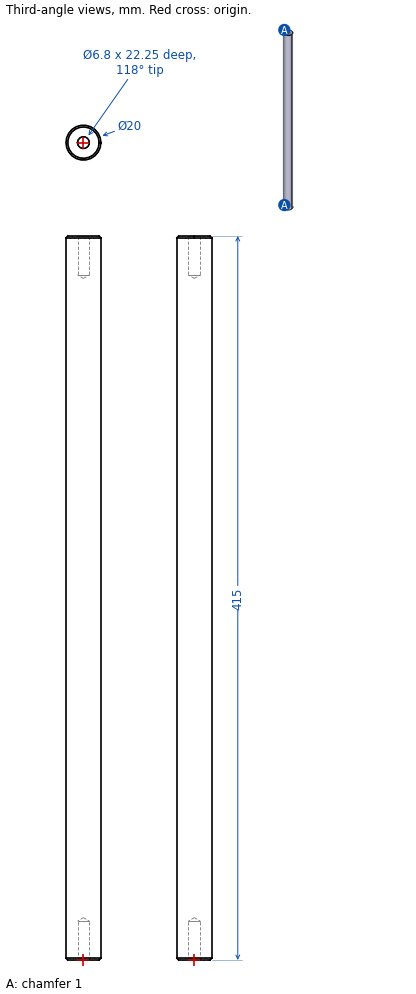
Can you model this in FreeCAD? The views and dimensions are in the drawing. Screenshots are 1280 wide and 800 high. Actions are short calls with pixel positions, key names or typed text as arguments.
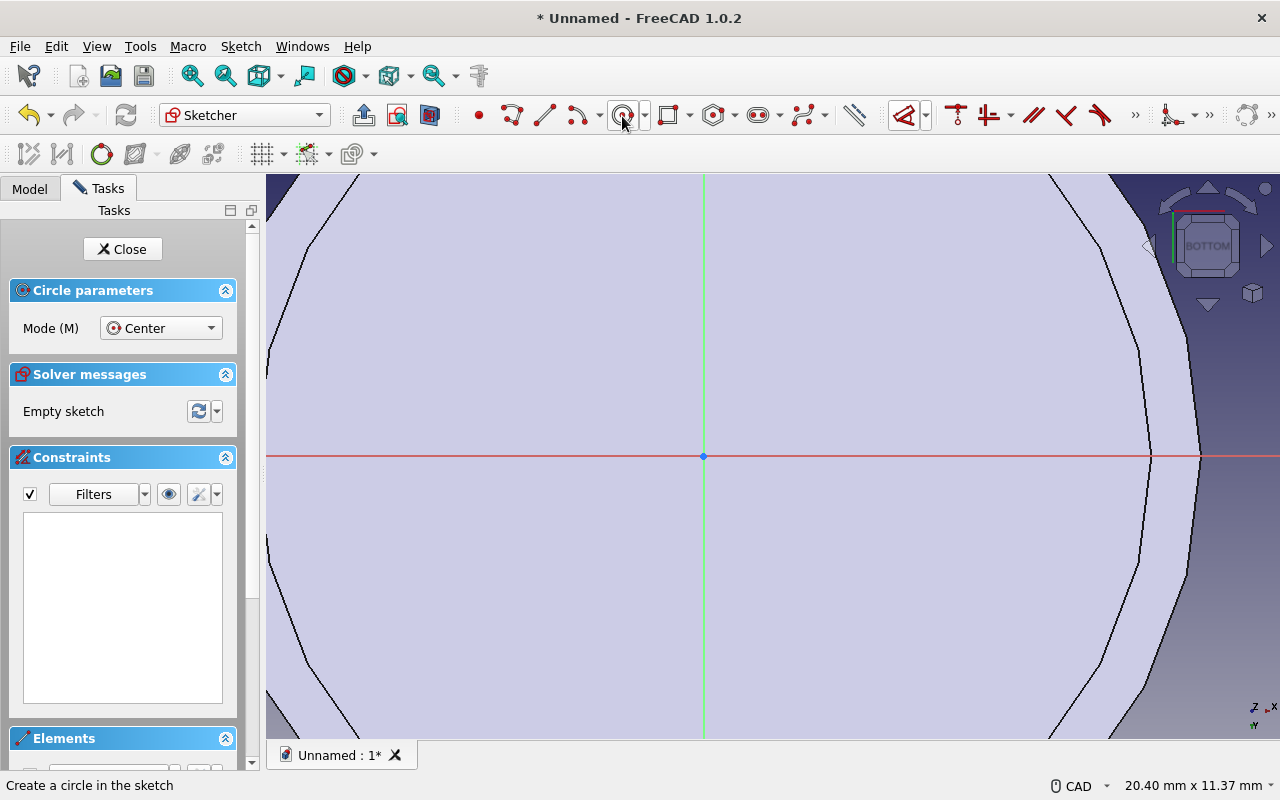
click(704, 456)
click(824, 337)
key(Escape)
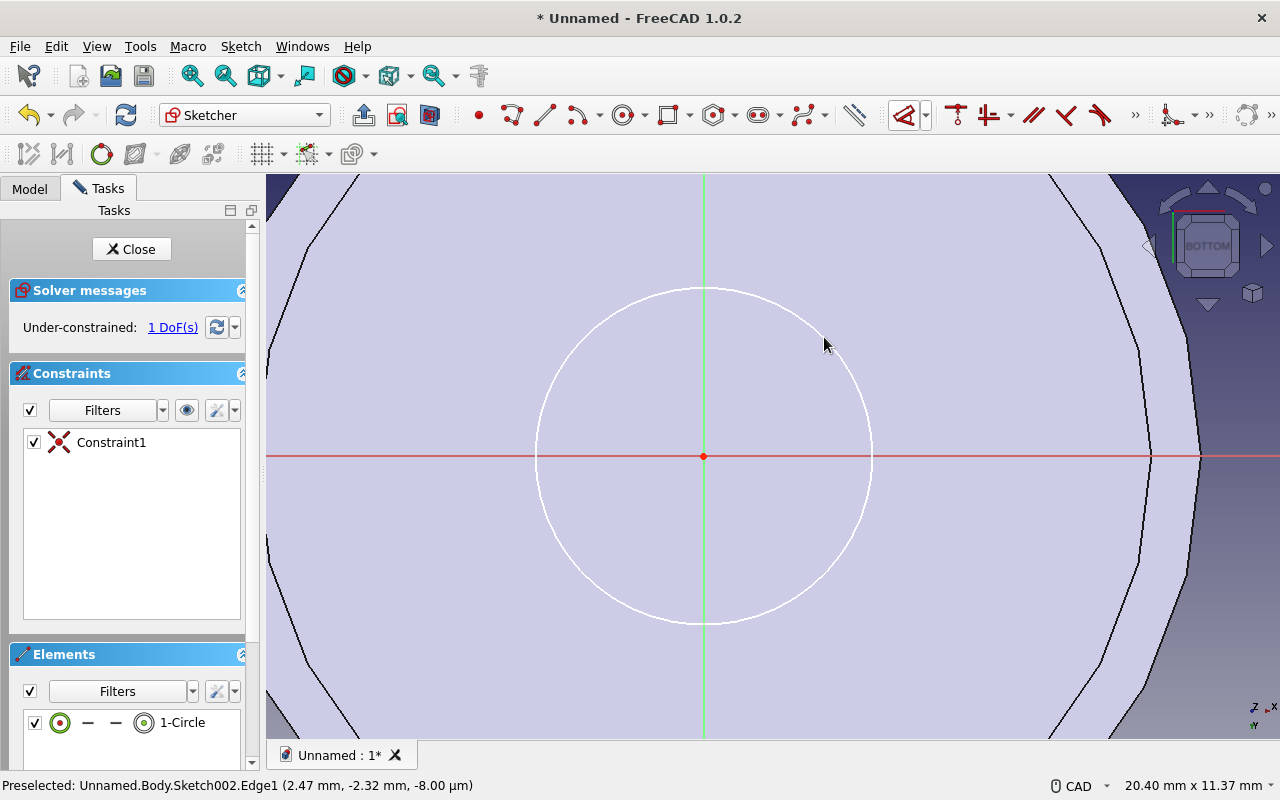
click(823, 337)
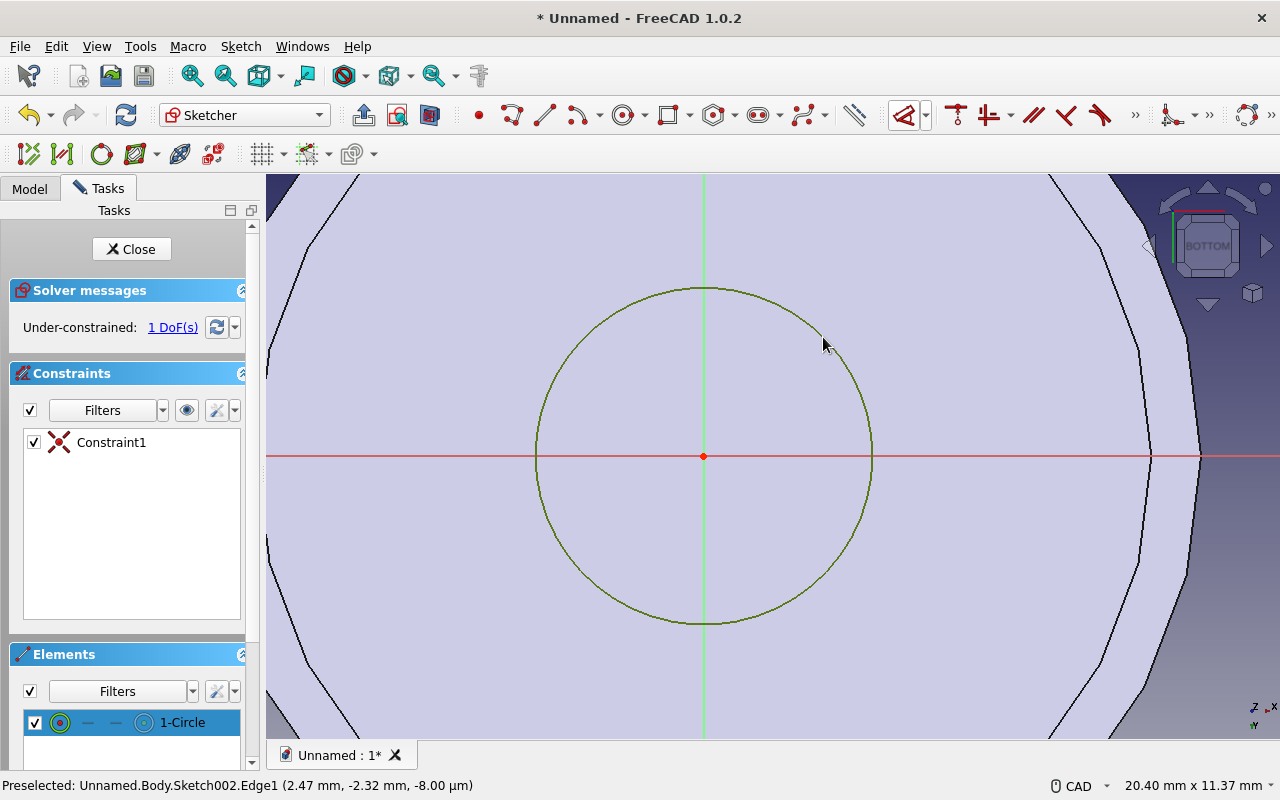
click(926, 116)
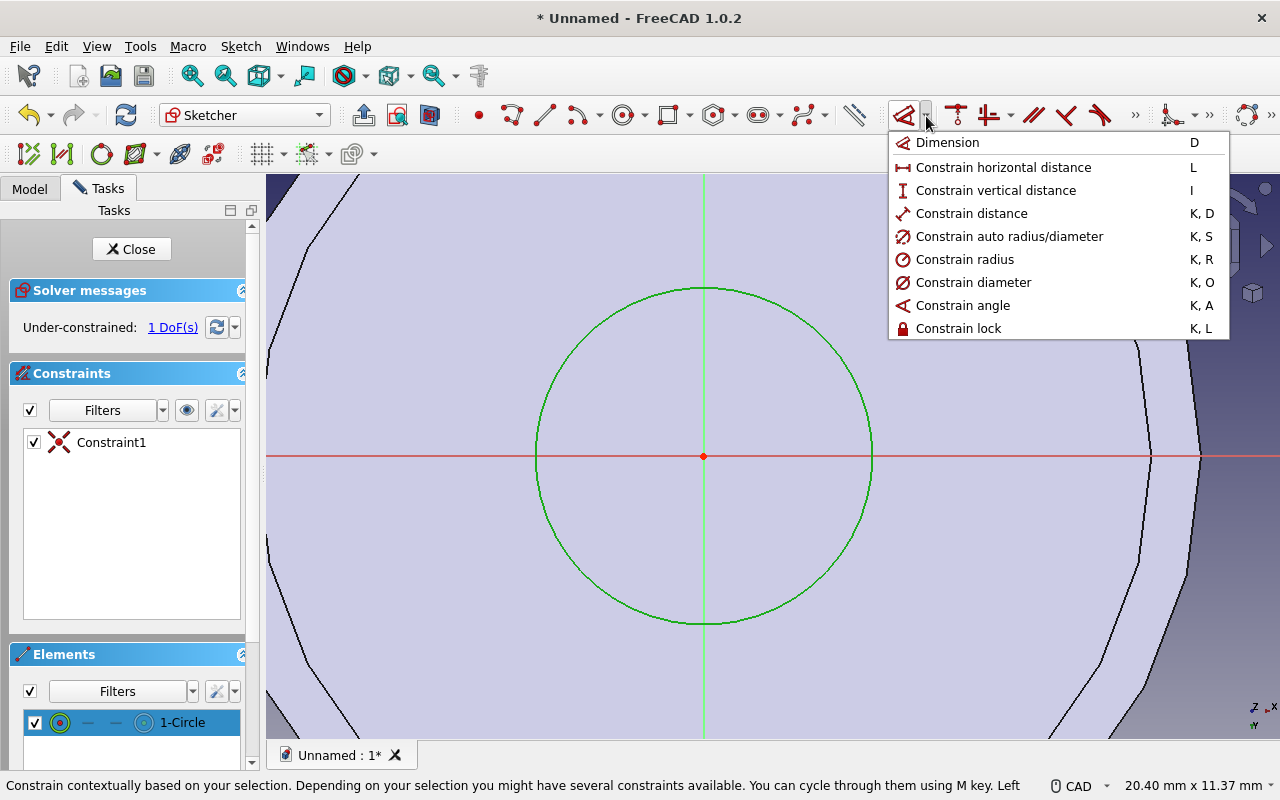
click(1059, 282)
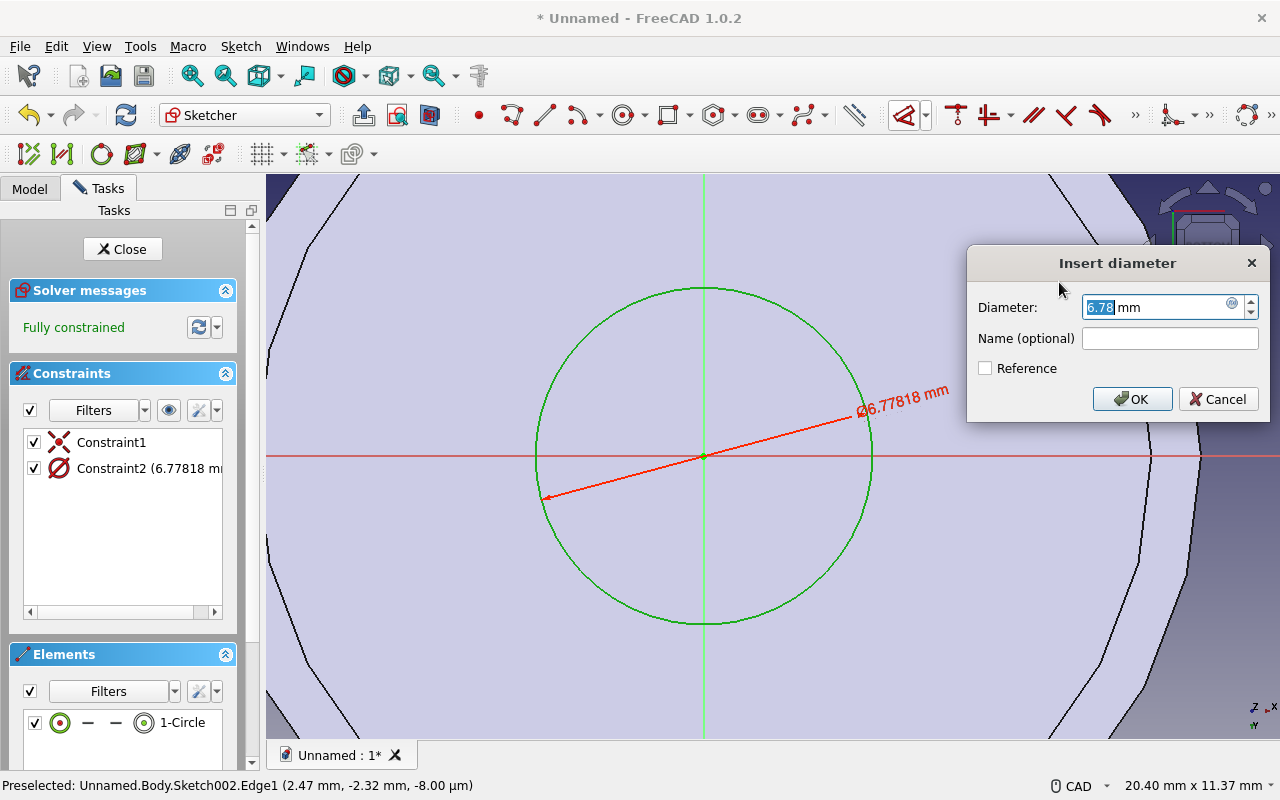
text(6.8)
key(Return)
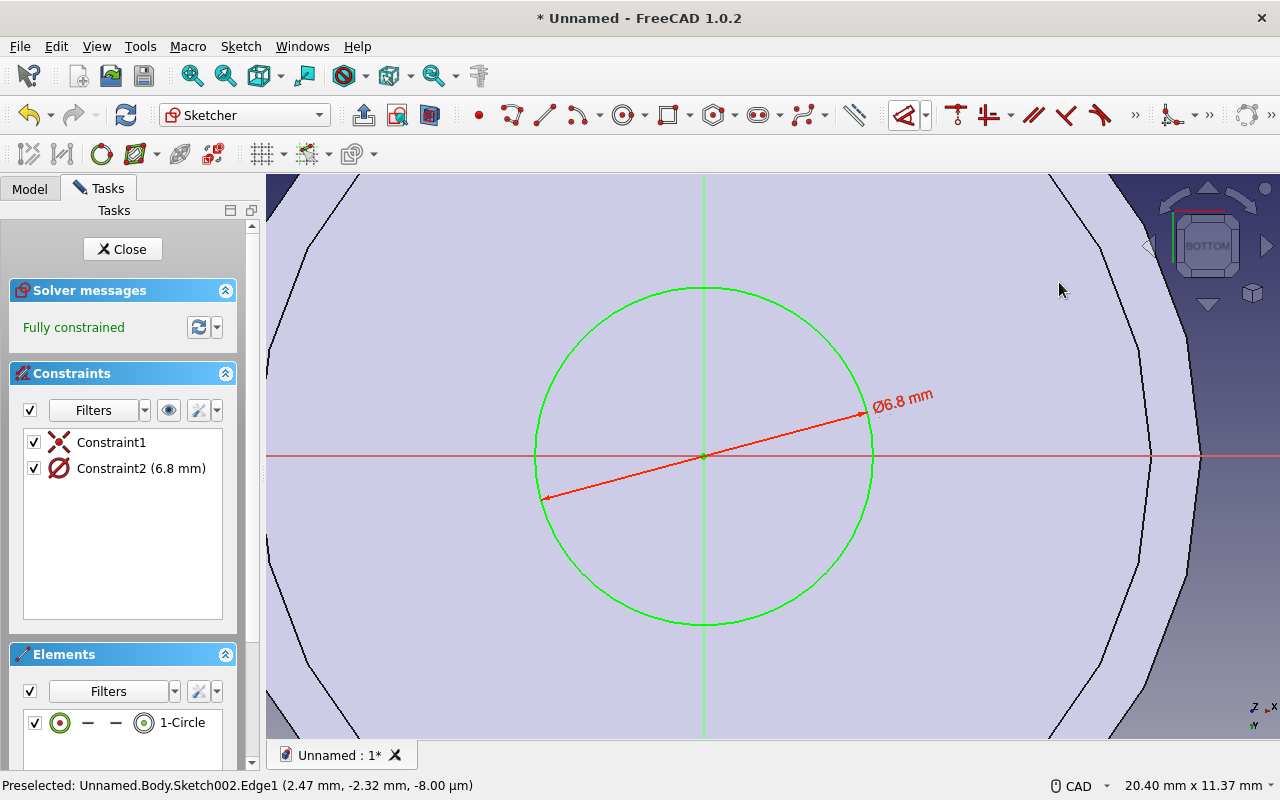
click(123, 249)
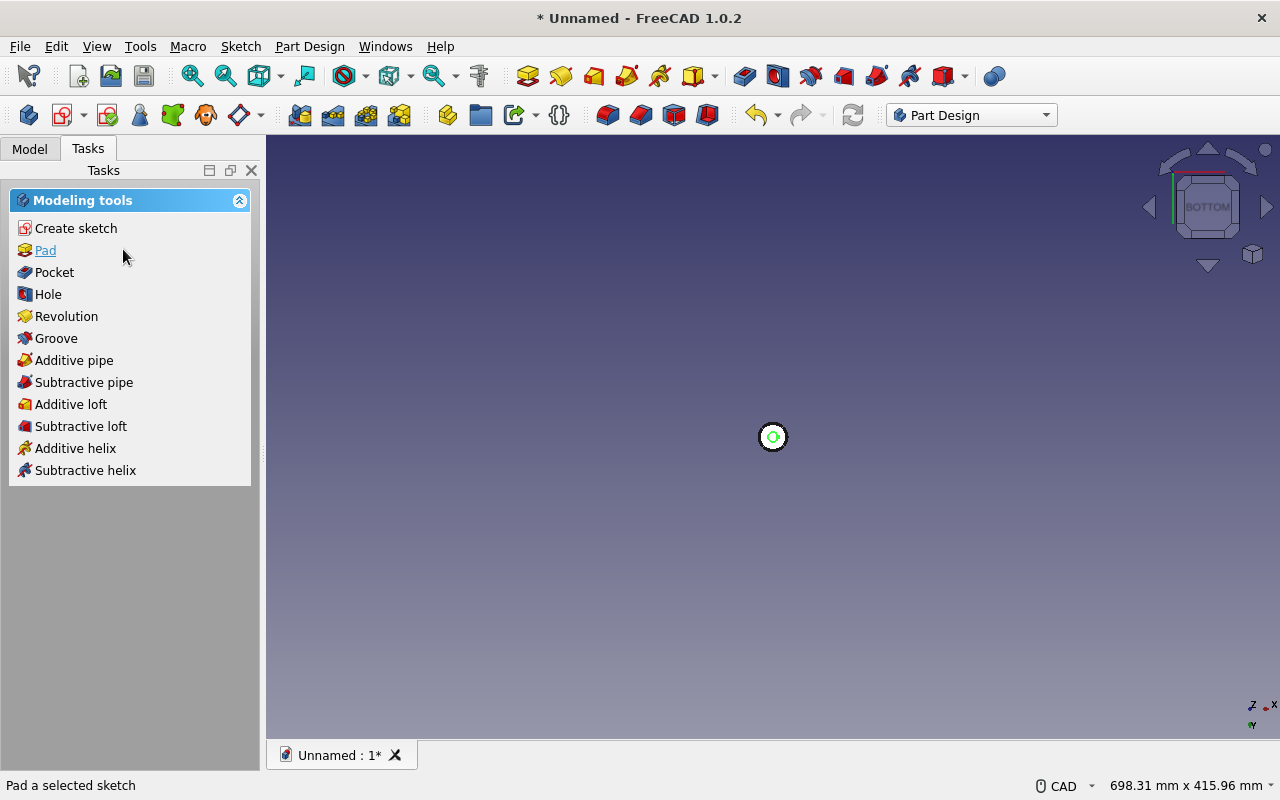
click(778, 76)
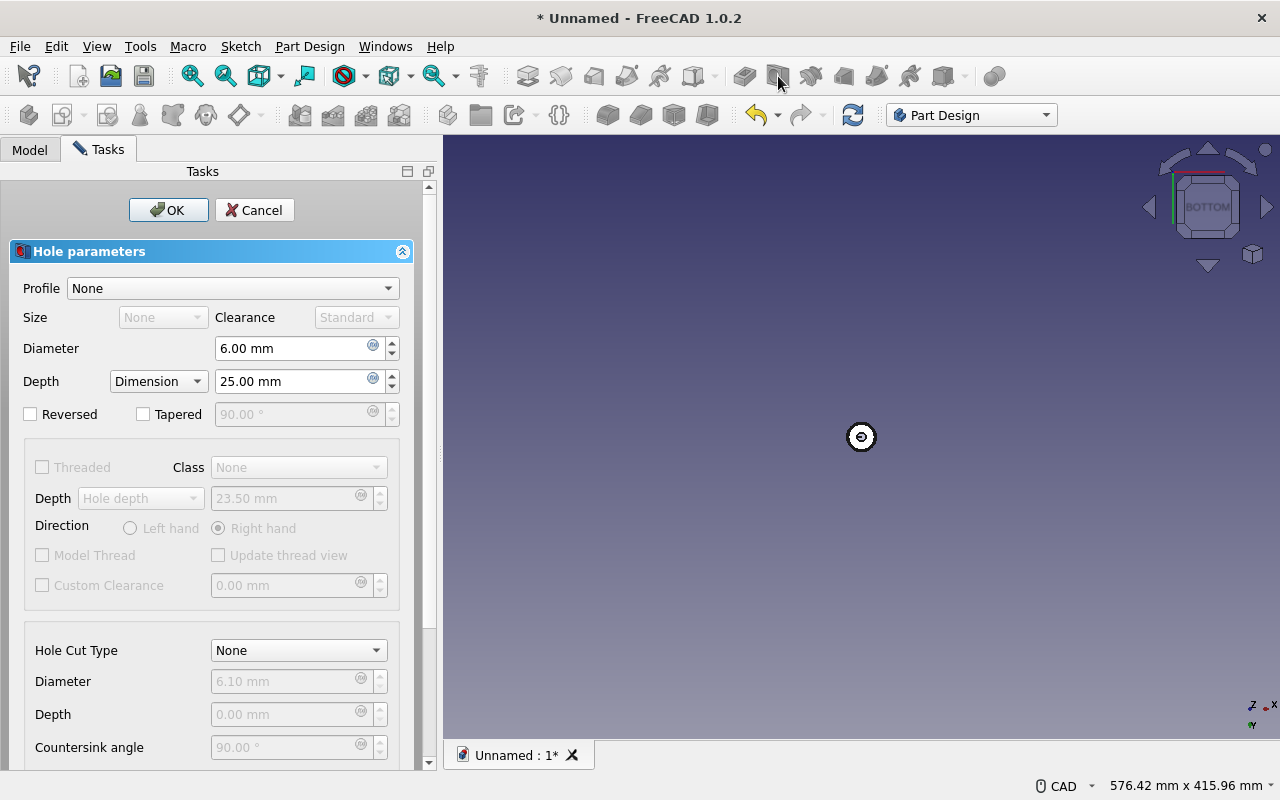
triple_click(300, 348)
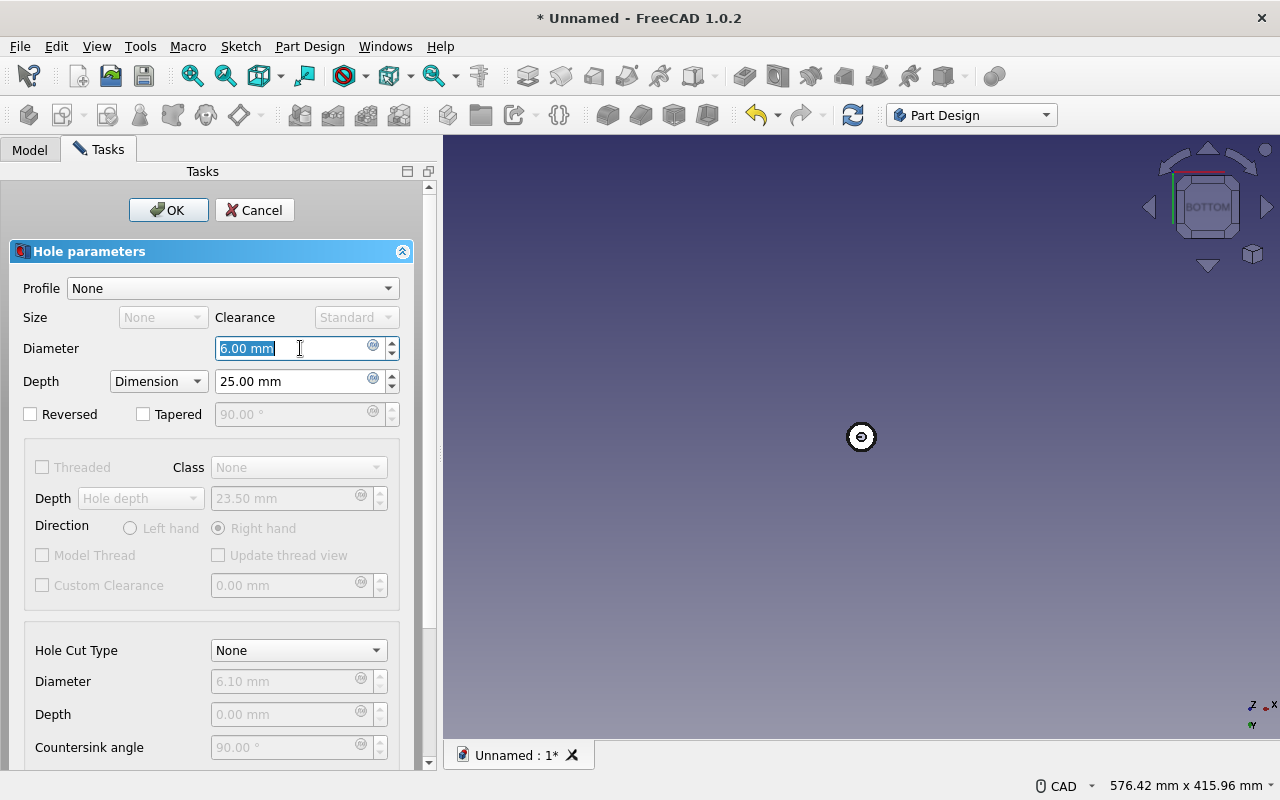
text(6.8)
key(Tab)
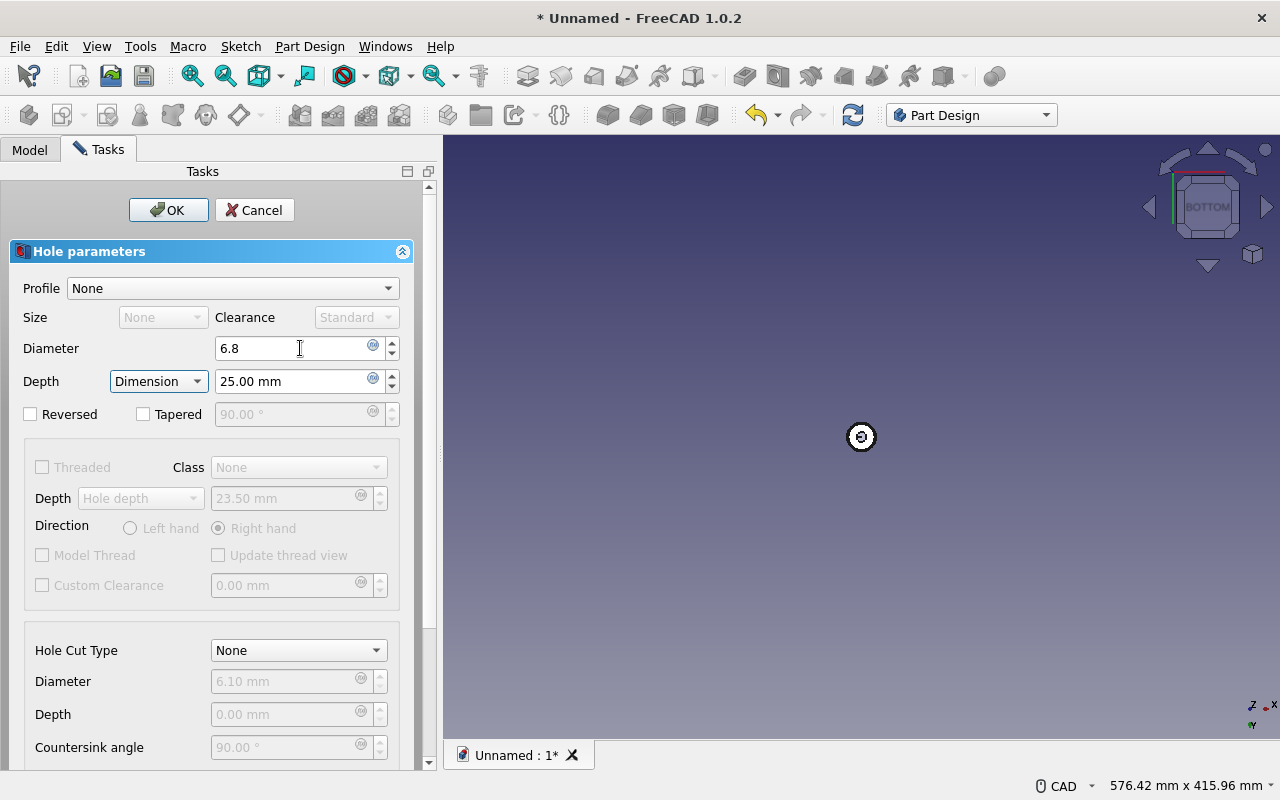
triple_click(300, 382)